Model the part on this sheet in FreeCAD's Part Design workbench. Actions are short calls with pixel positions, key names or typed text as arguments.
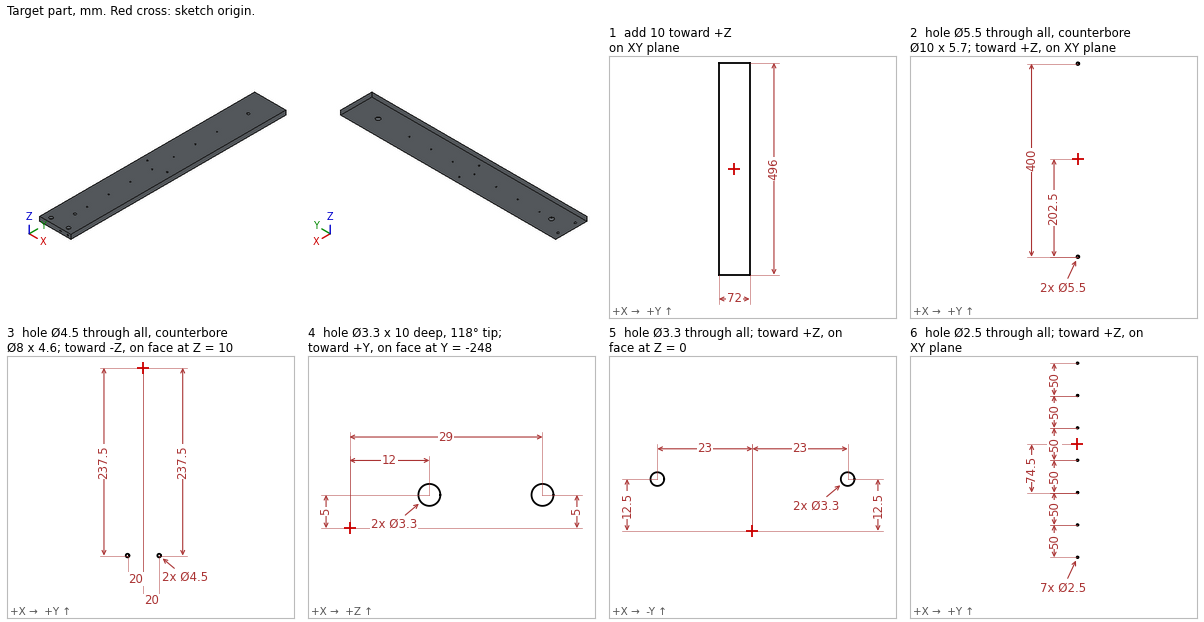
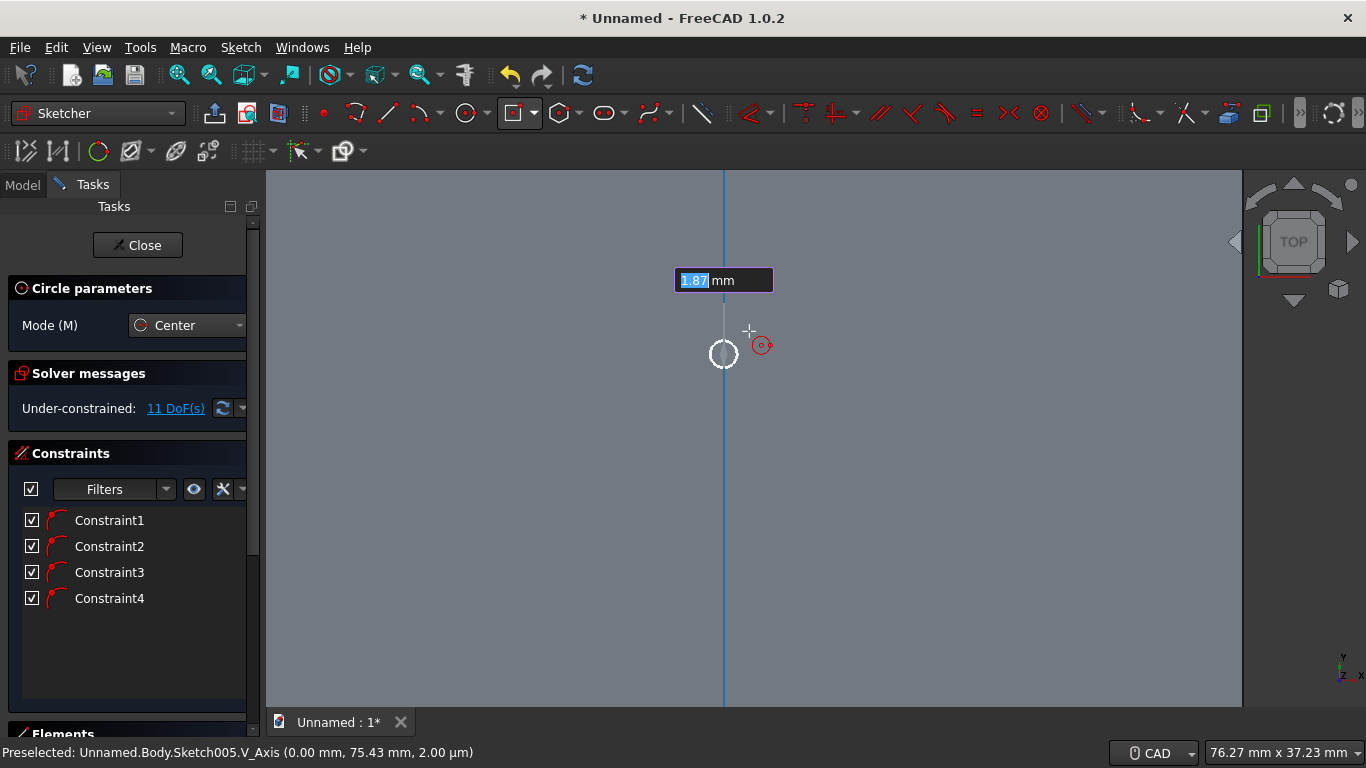
click(741, 333)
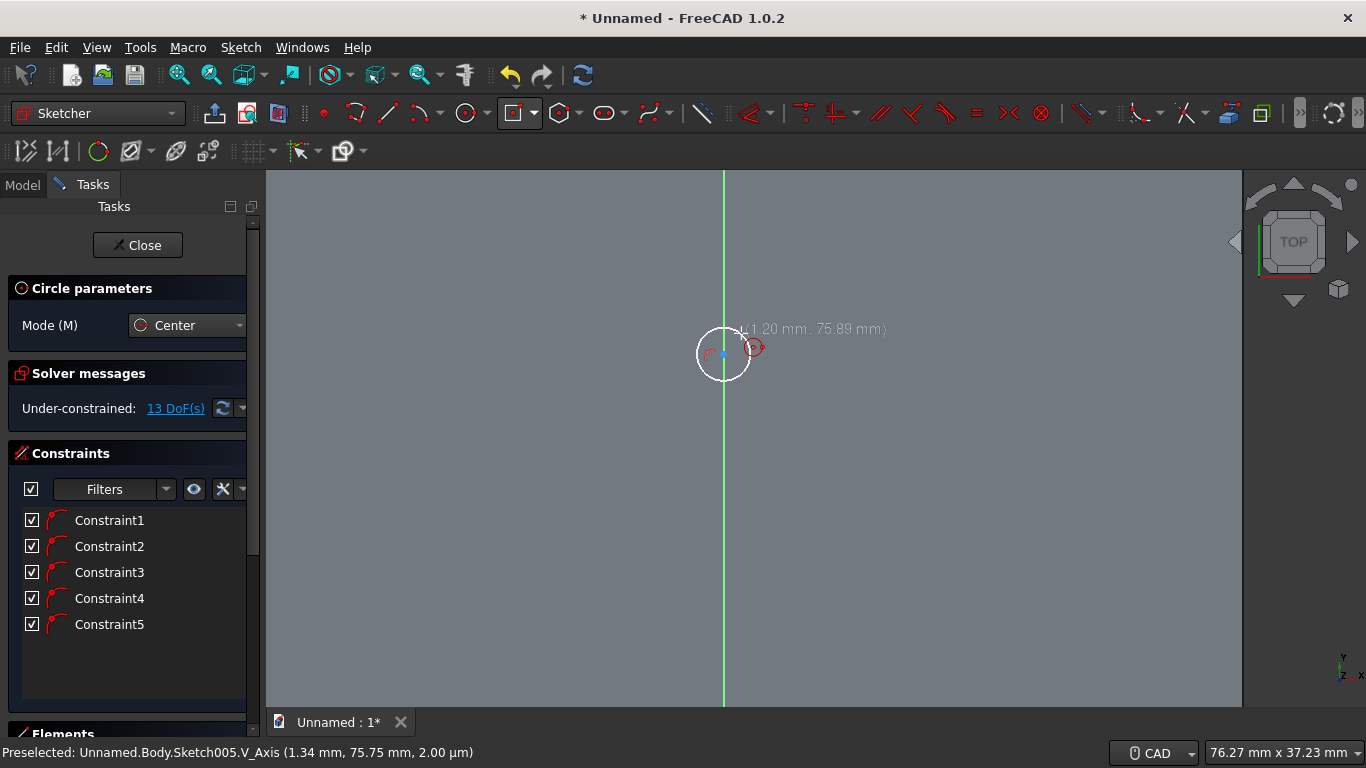
scroll(749, 331, down, 13)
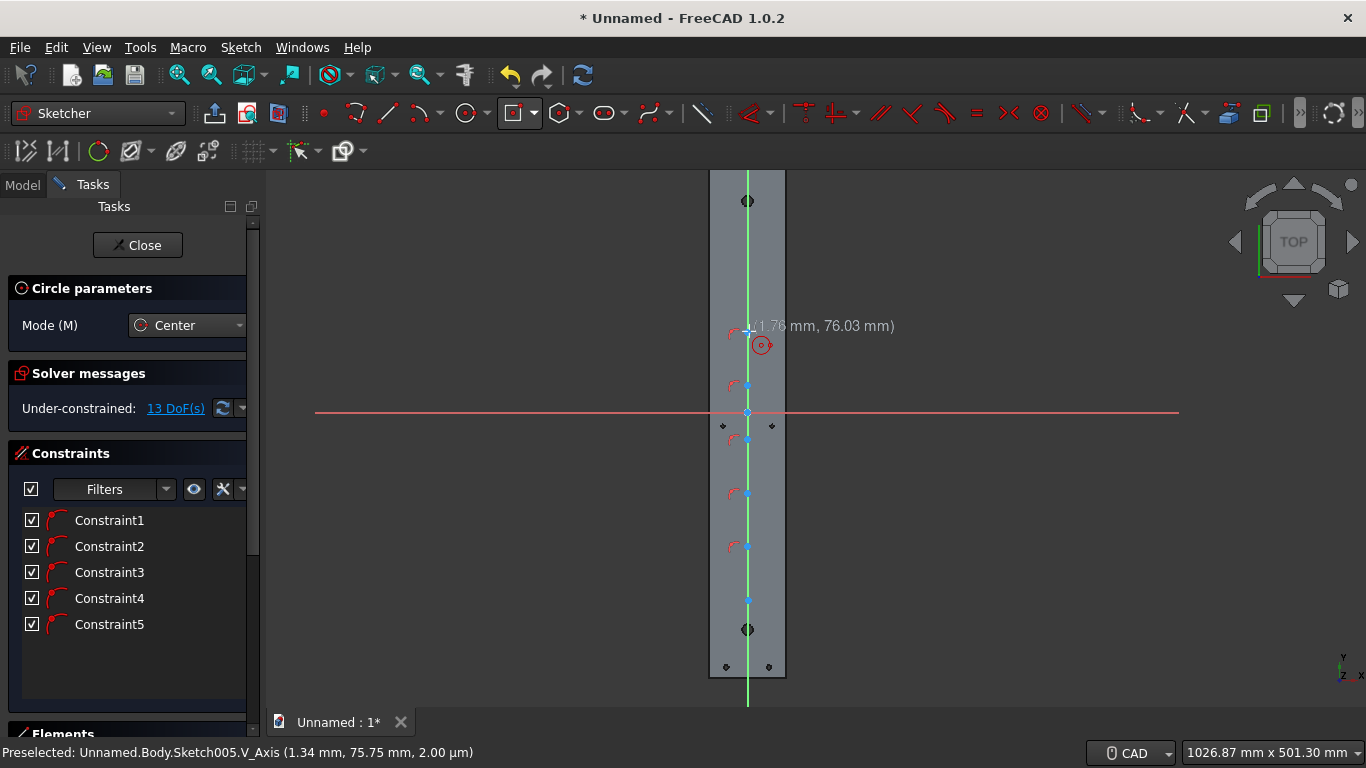
scroll(748, 278, up, 15)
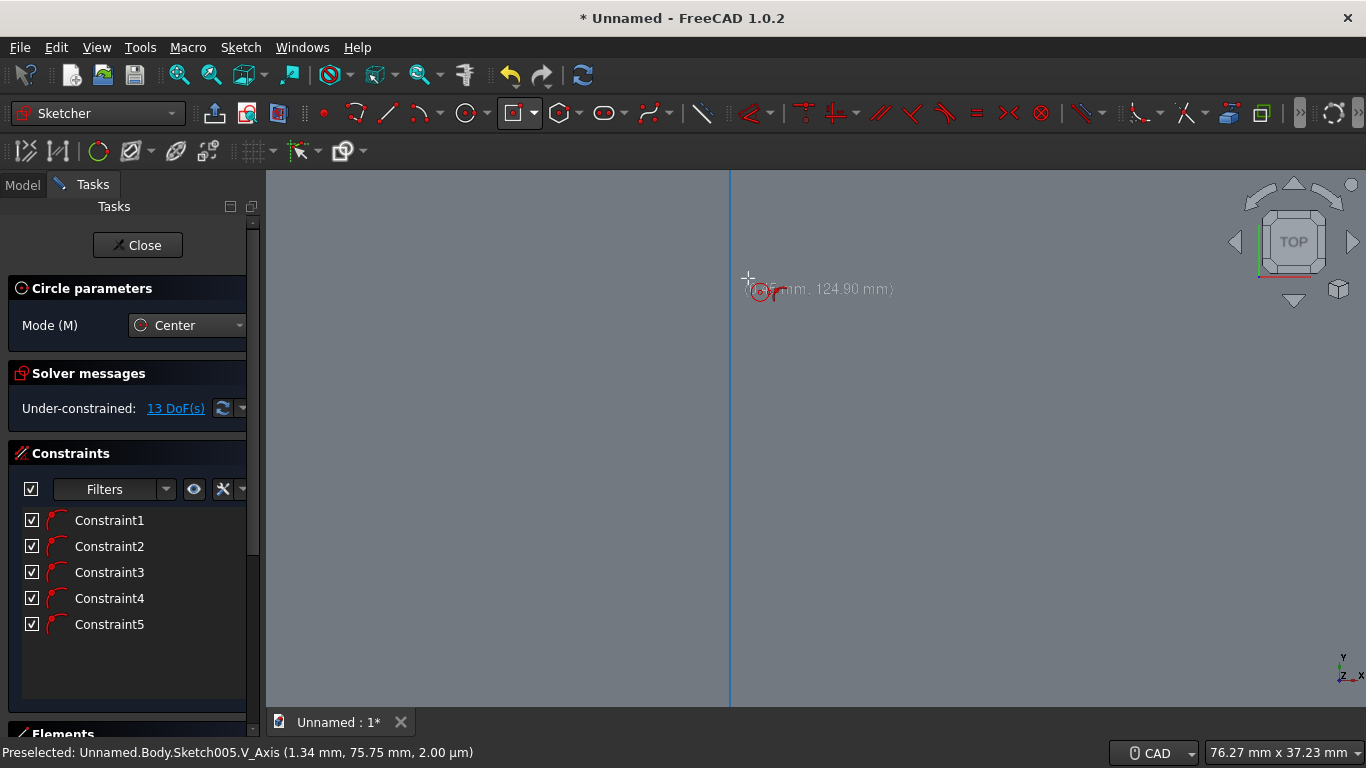
scroll(748, 278, down, 15)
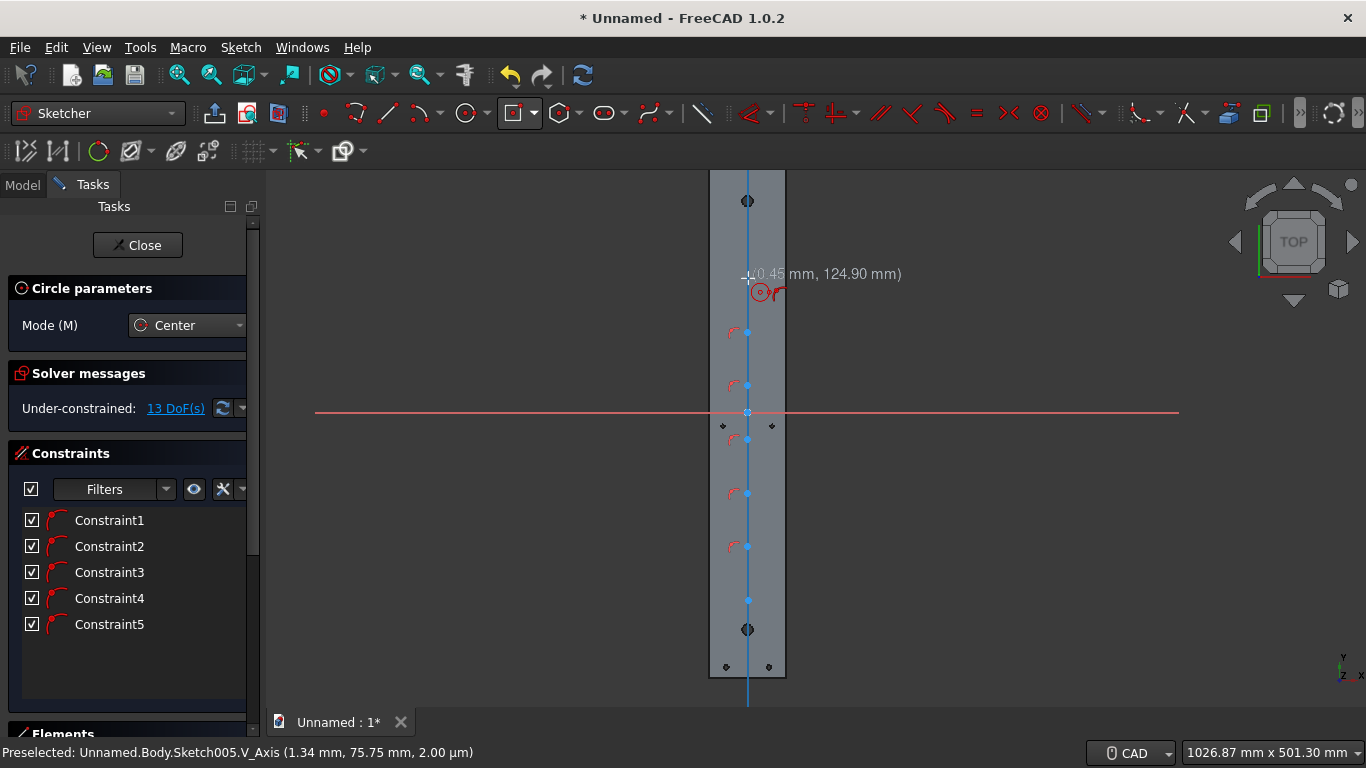
click(748, 278)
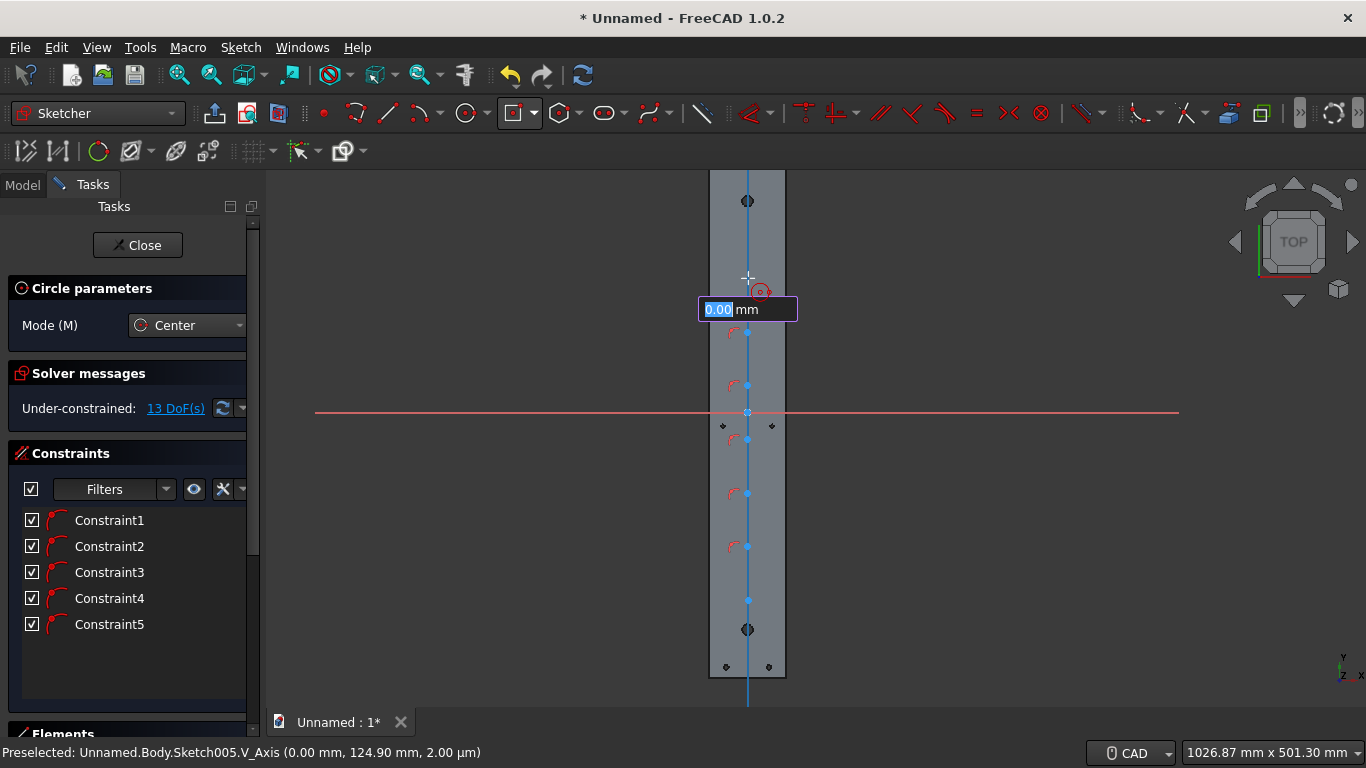
scroll(749, 278, up, 13)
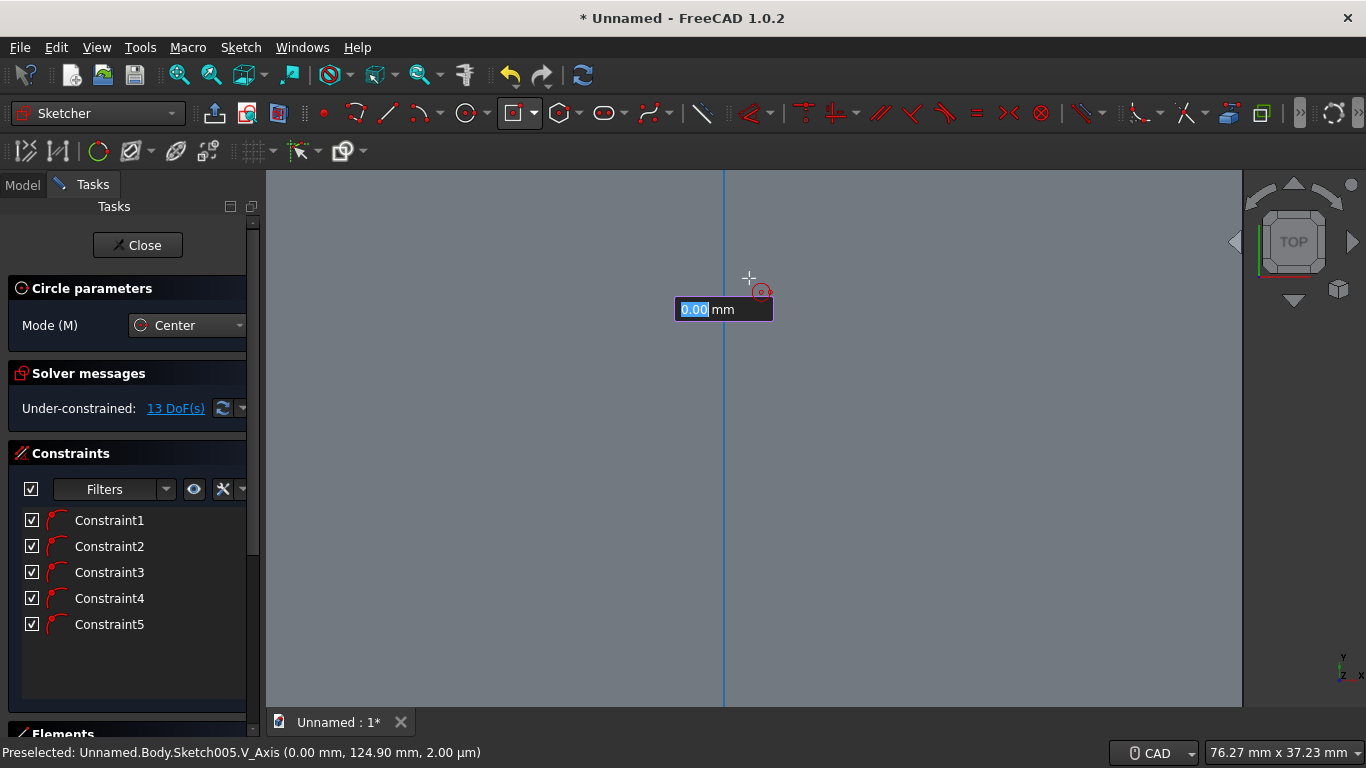
click(741, 274)
key(Escape)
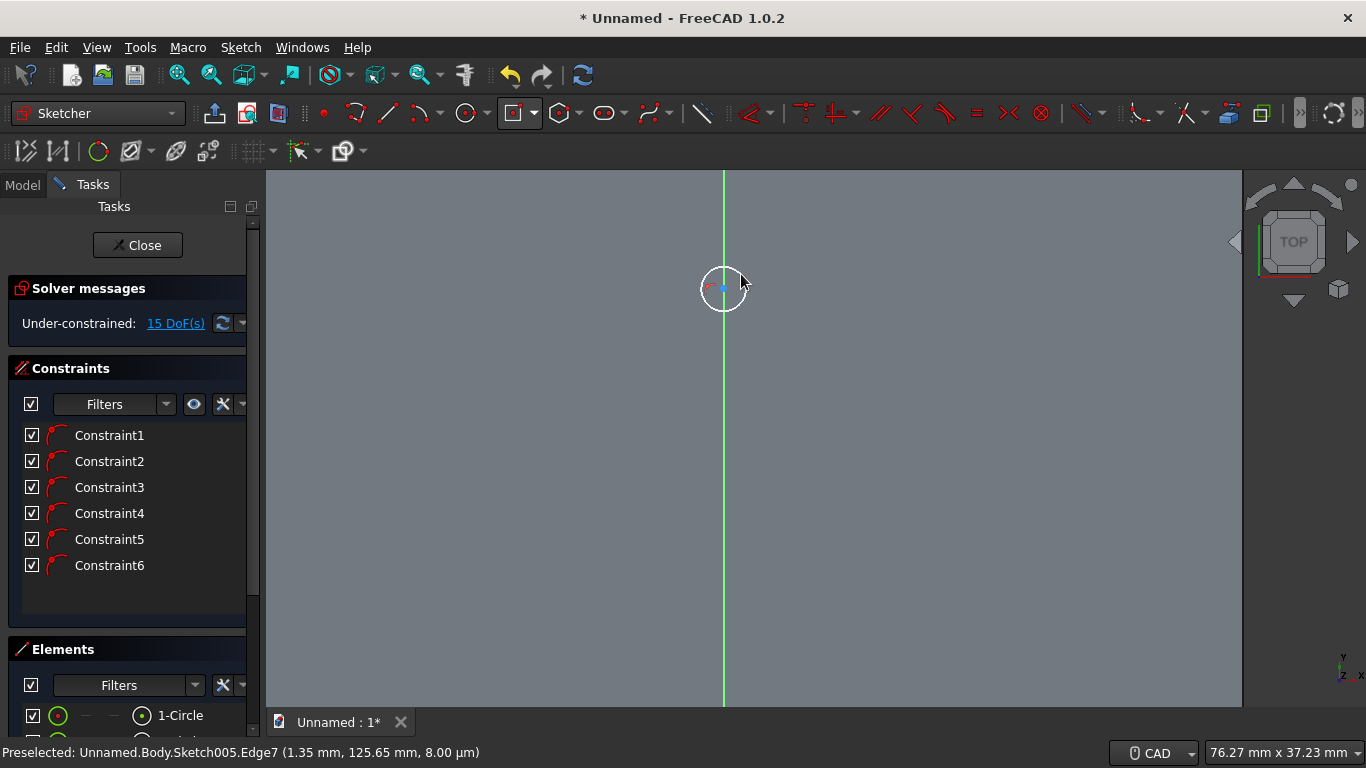
scroll(749, 278, down, 13)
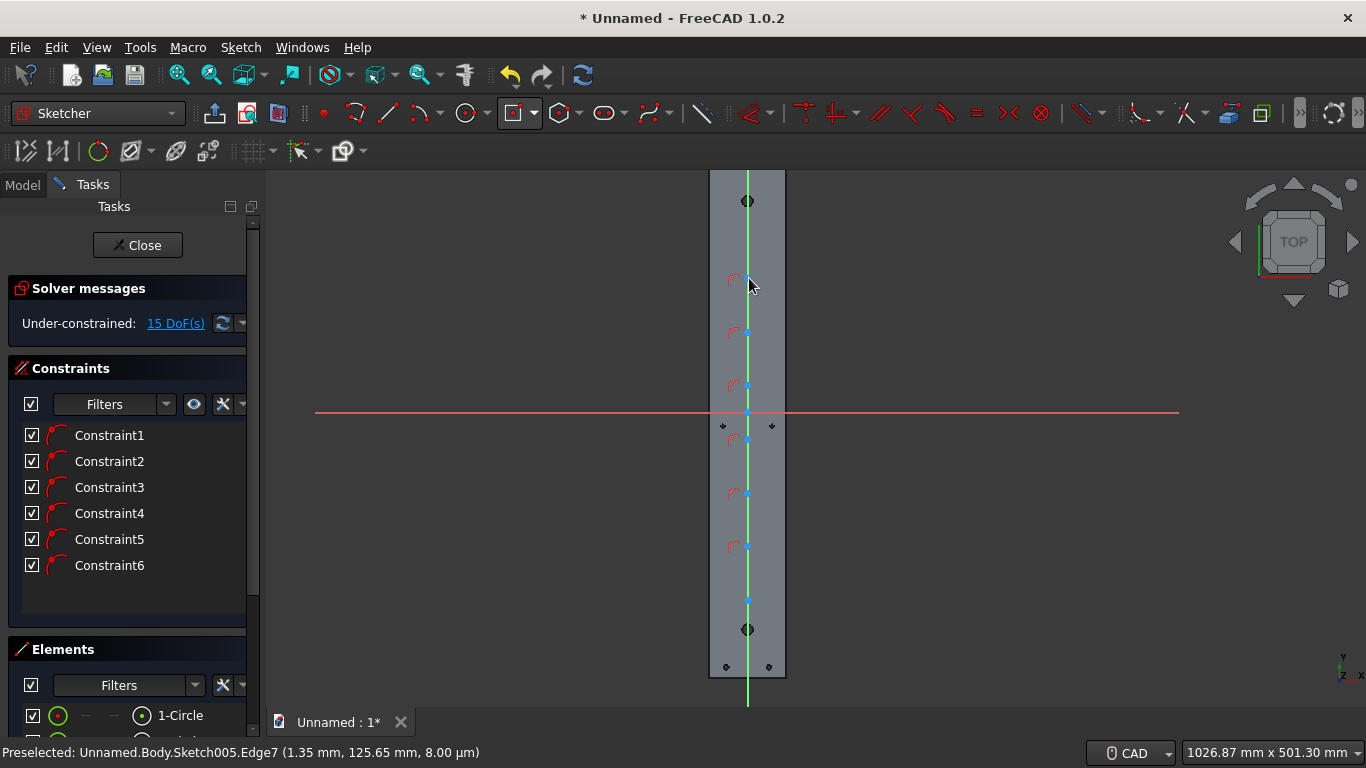
scroll(749, 600, up, 11)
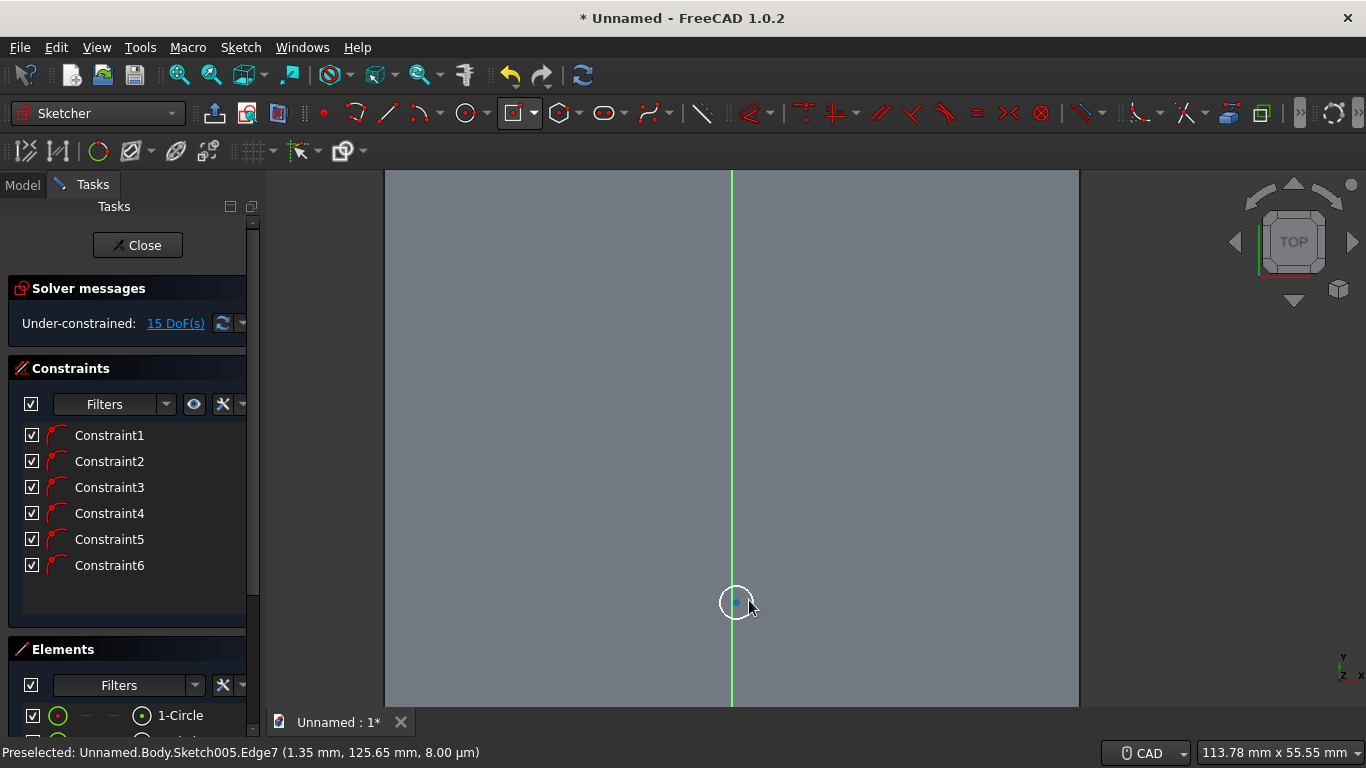
click(748, 591)